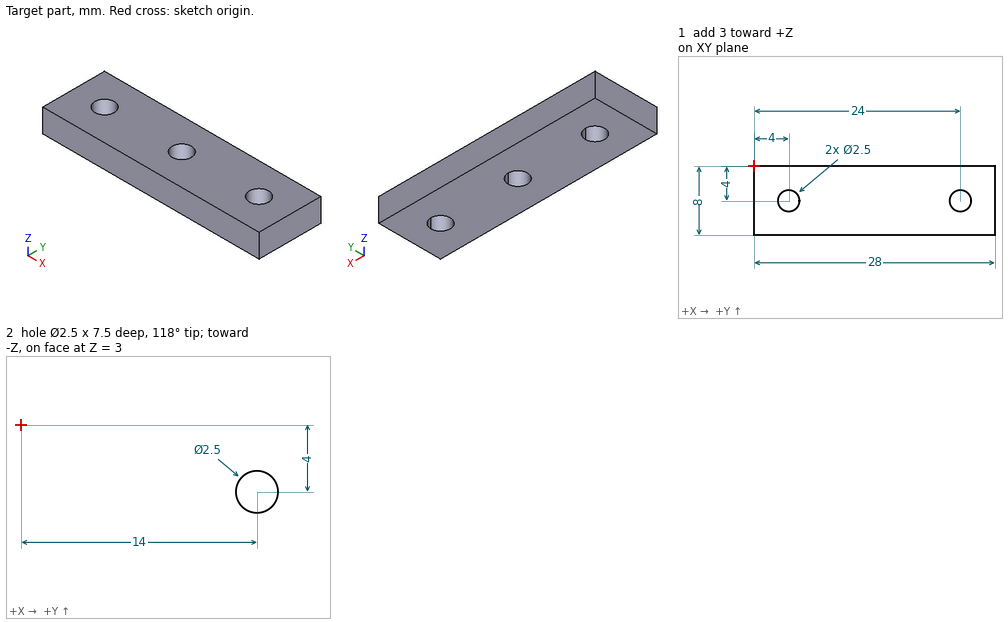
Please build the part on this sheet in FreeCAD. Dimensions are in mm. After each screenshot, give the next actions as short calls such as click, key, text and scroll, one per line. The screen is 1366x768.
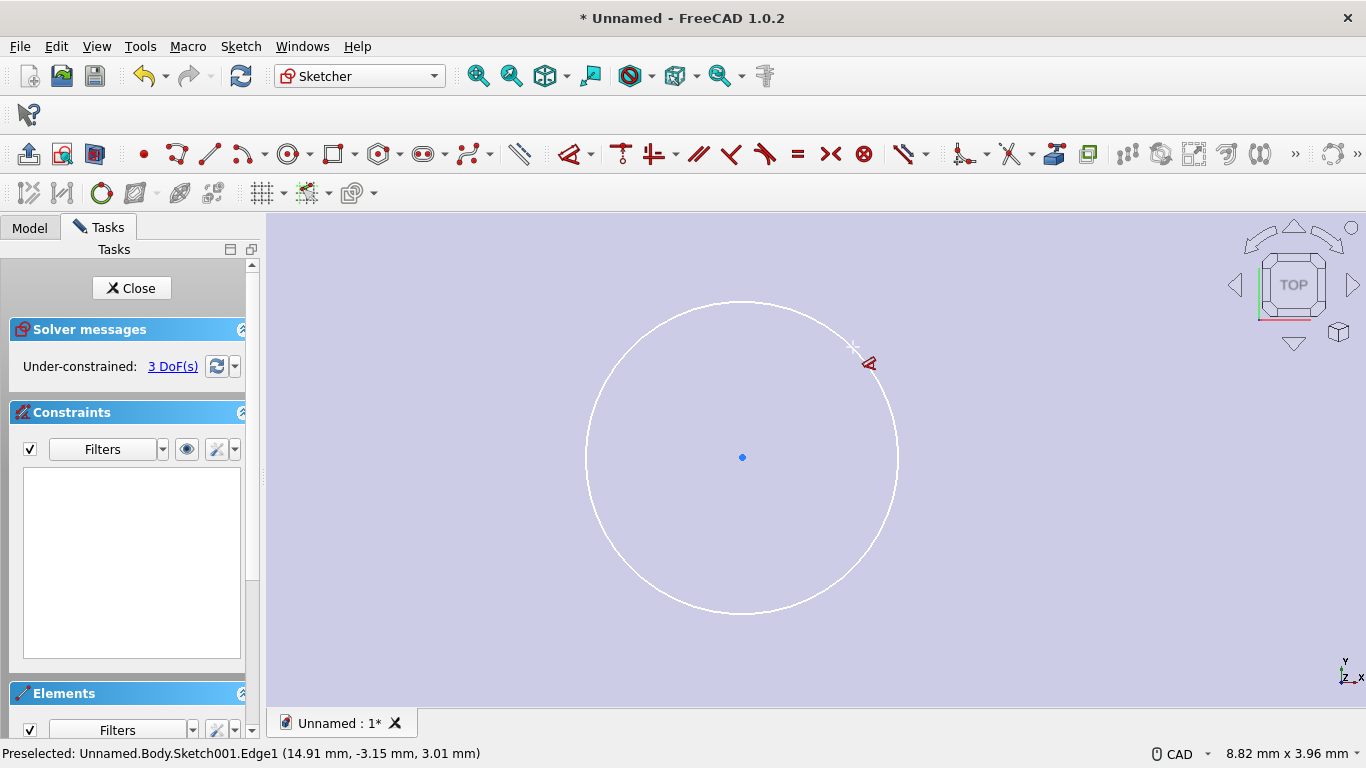
click(852, 347)
click(875, 324)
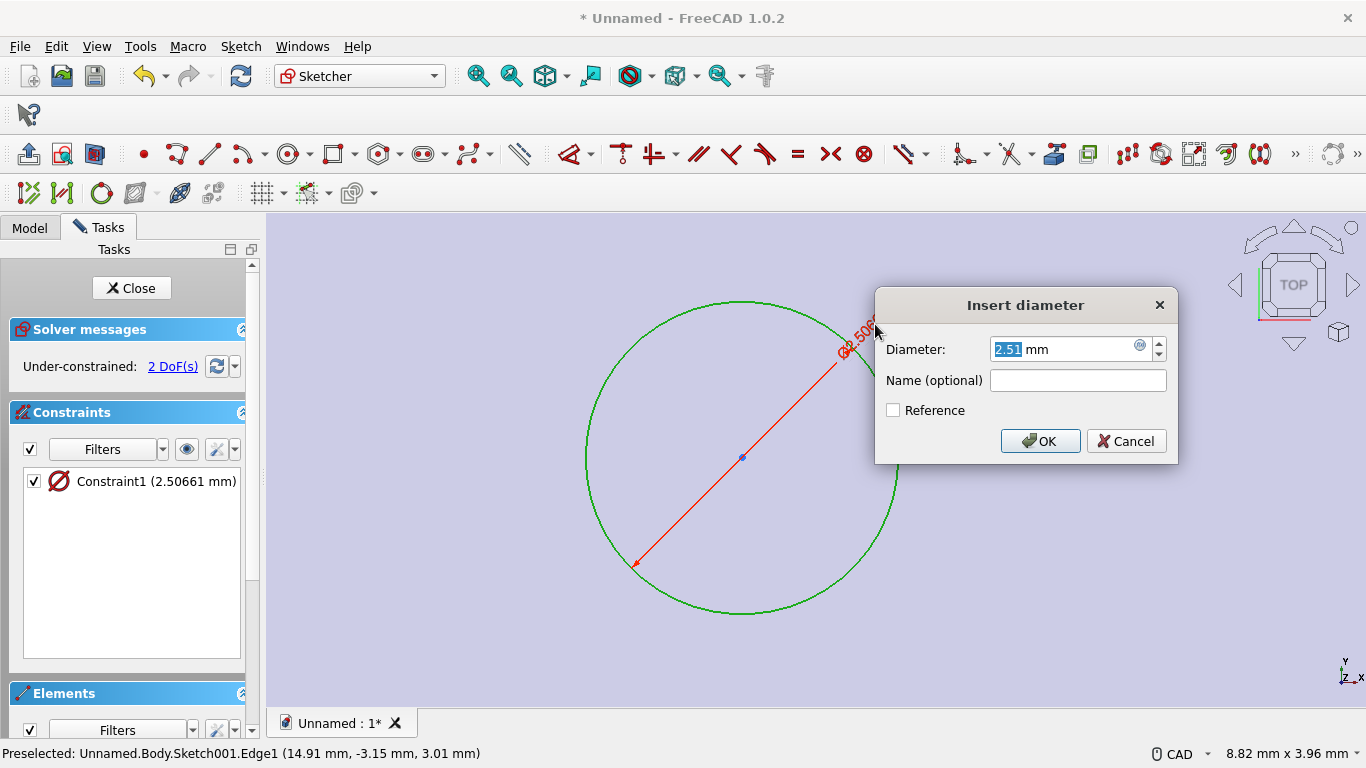
text(2.5)
key(Return)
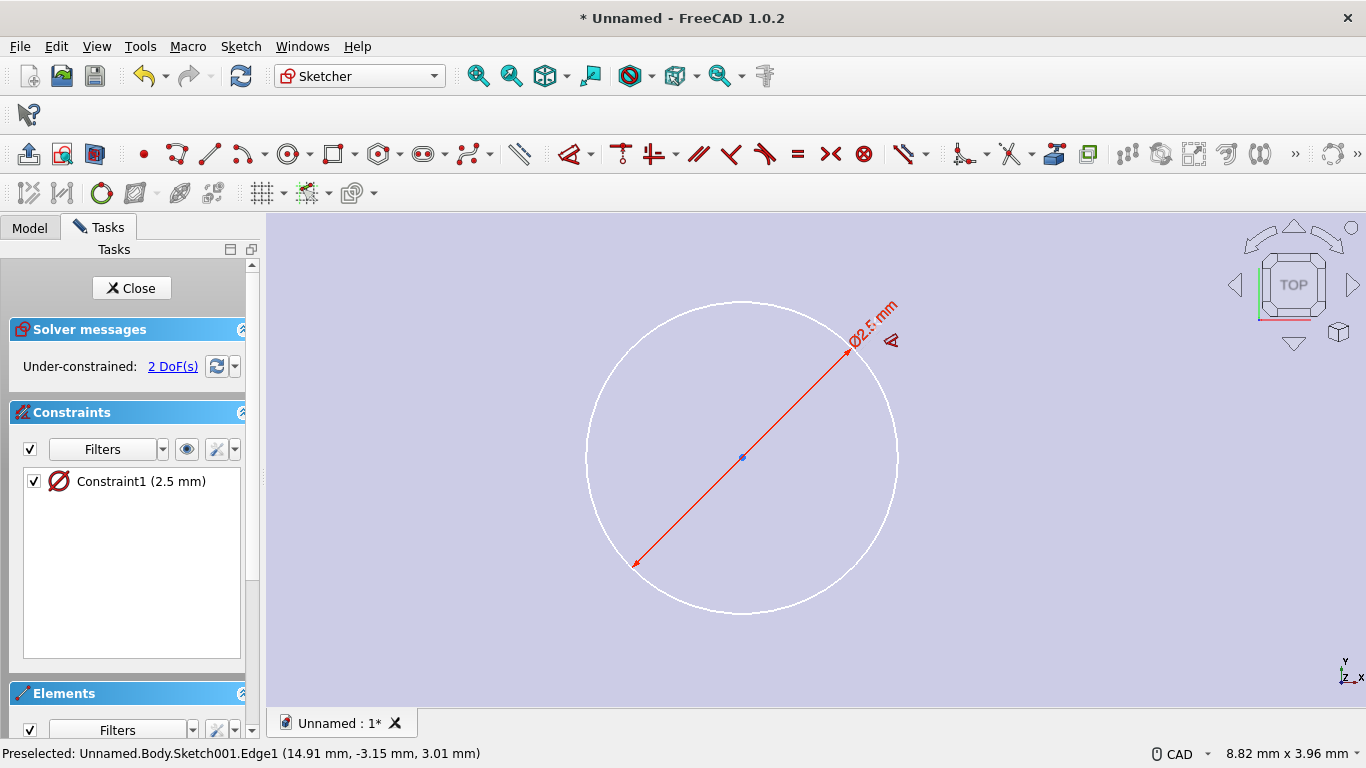
click(742, 458)
click(776, 350)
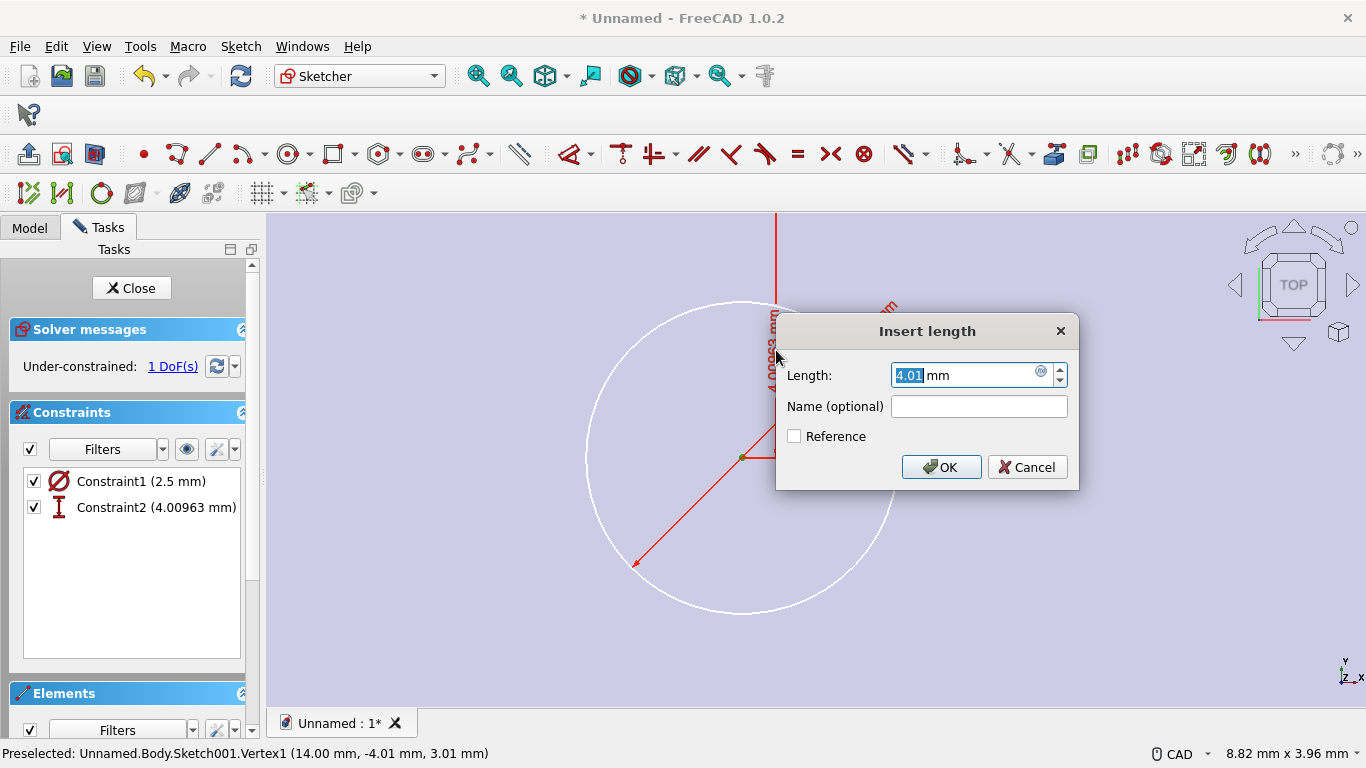
text(4)
key(Return)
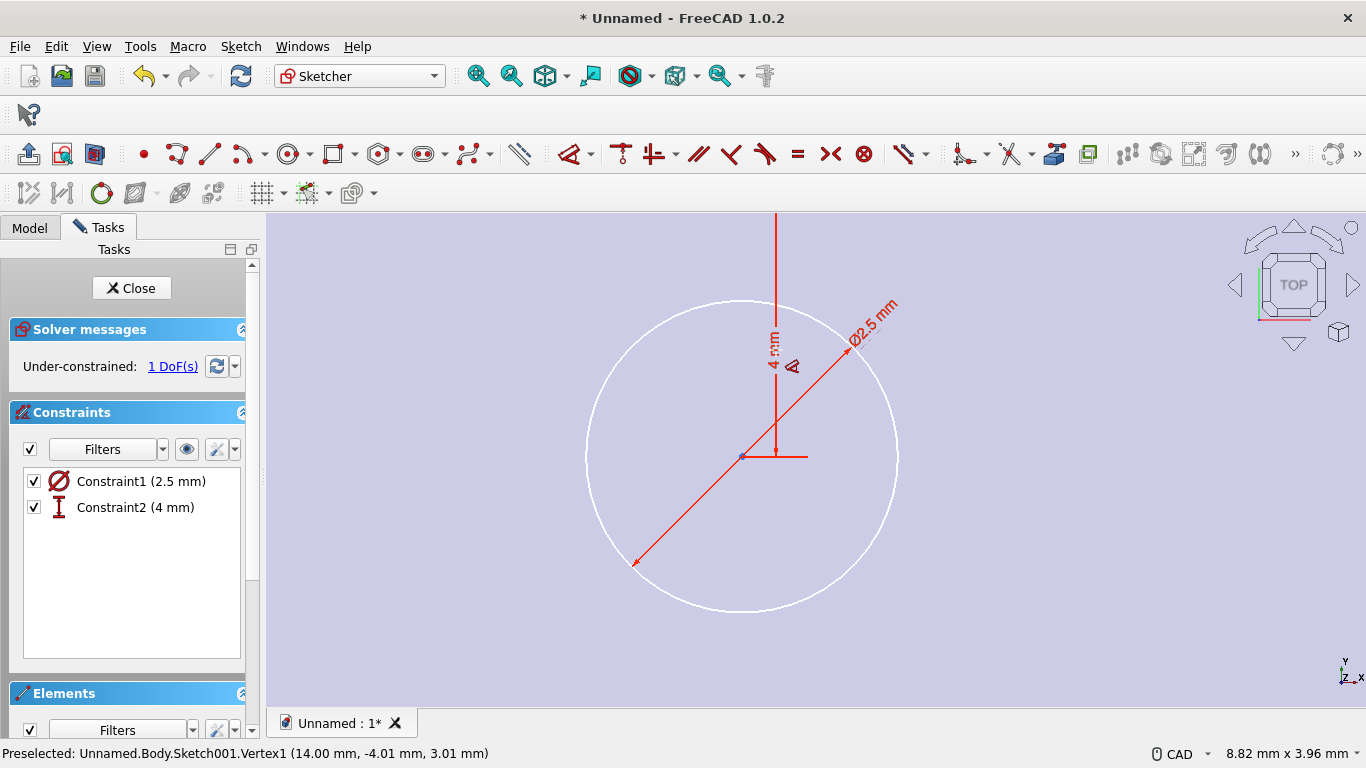
click(742, 457)
click(518, 491)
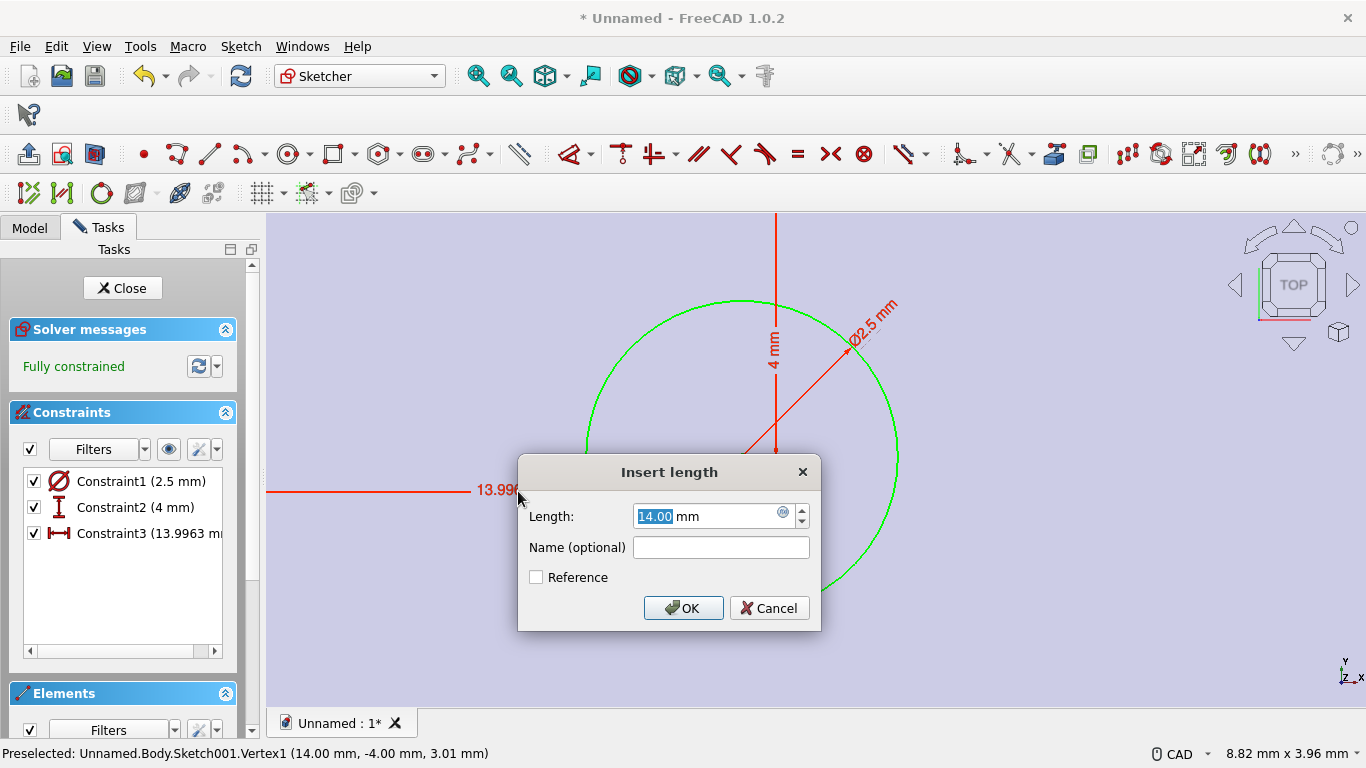
text(14)
key(Return)
key(Escape)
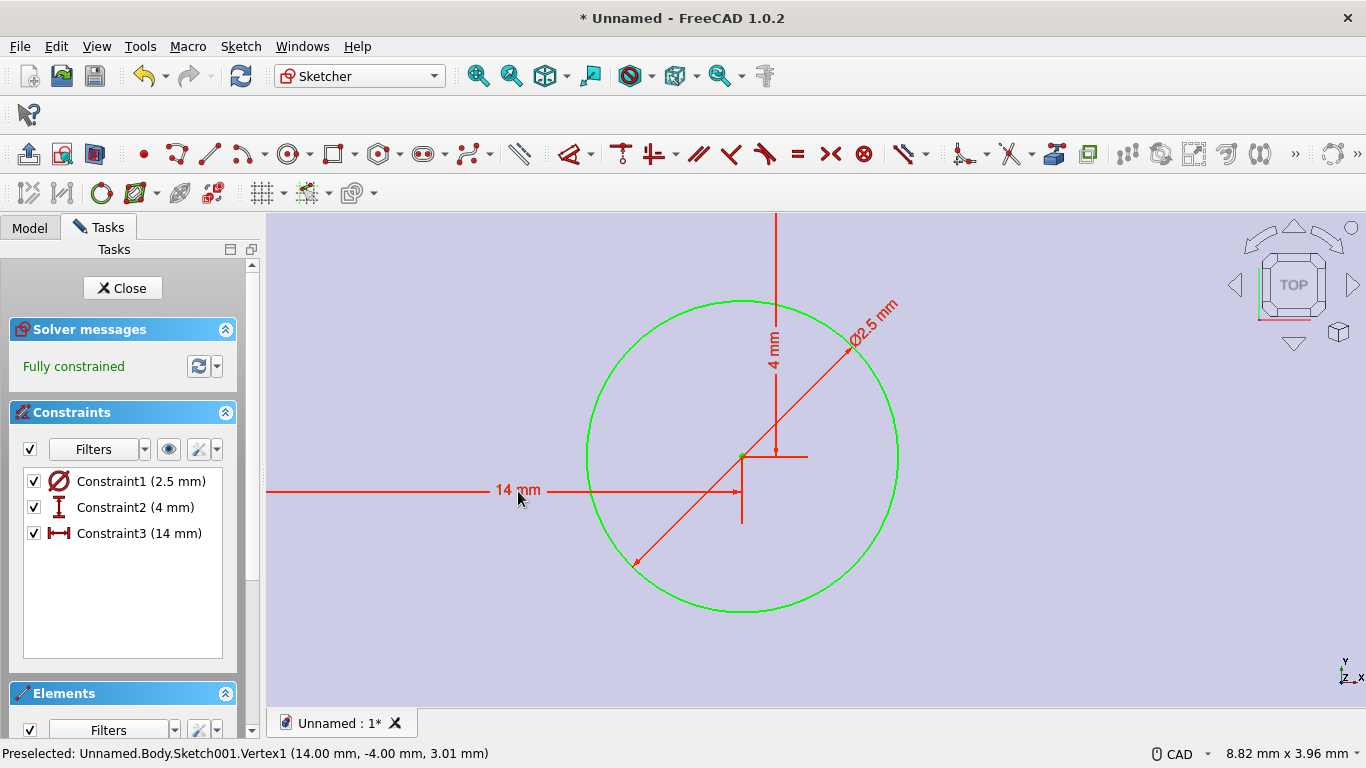
click(123, 288)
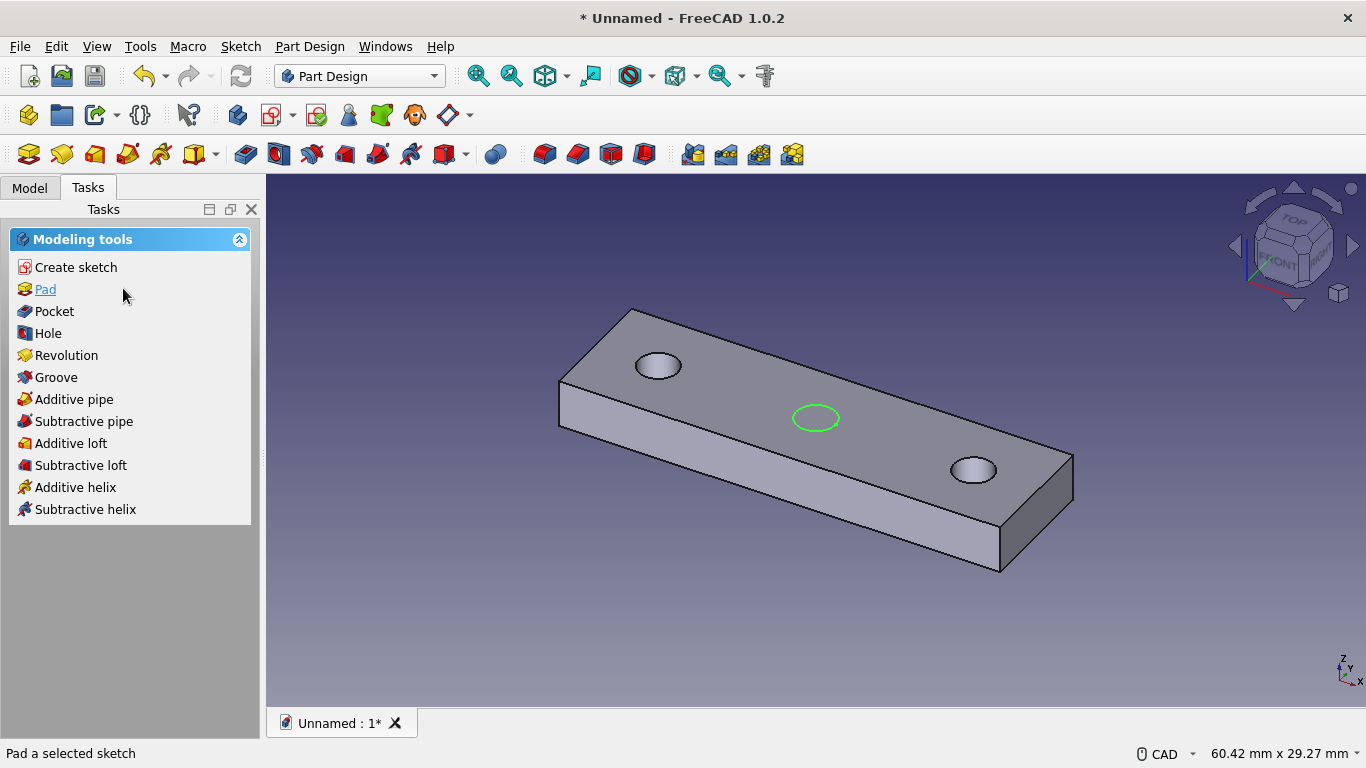
click(279, 154)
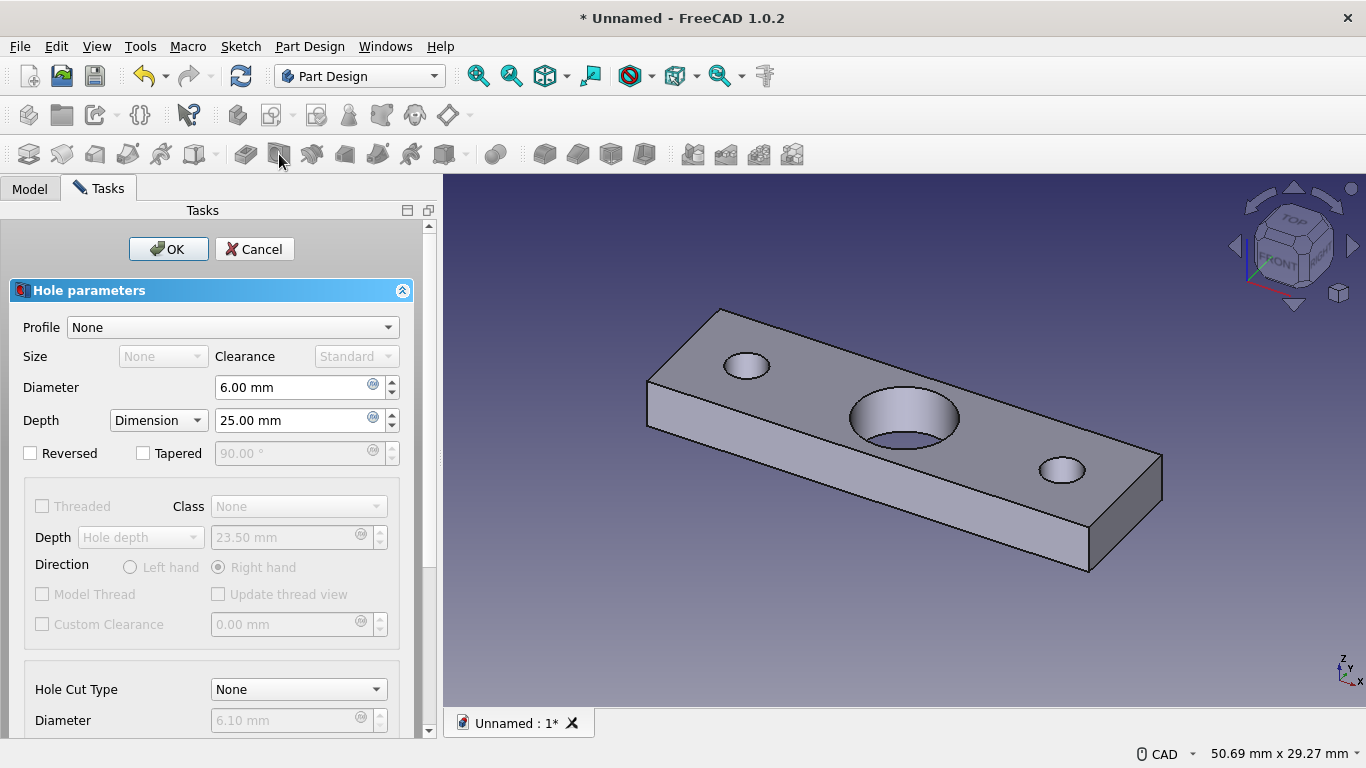
triple_click(300, 388)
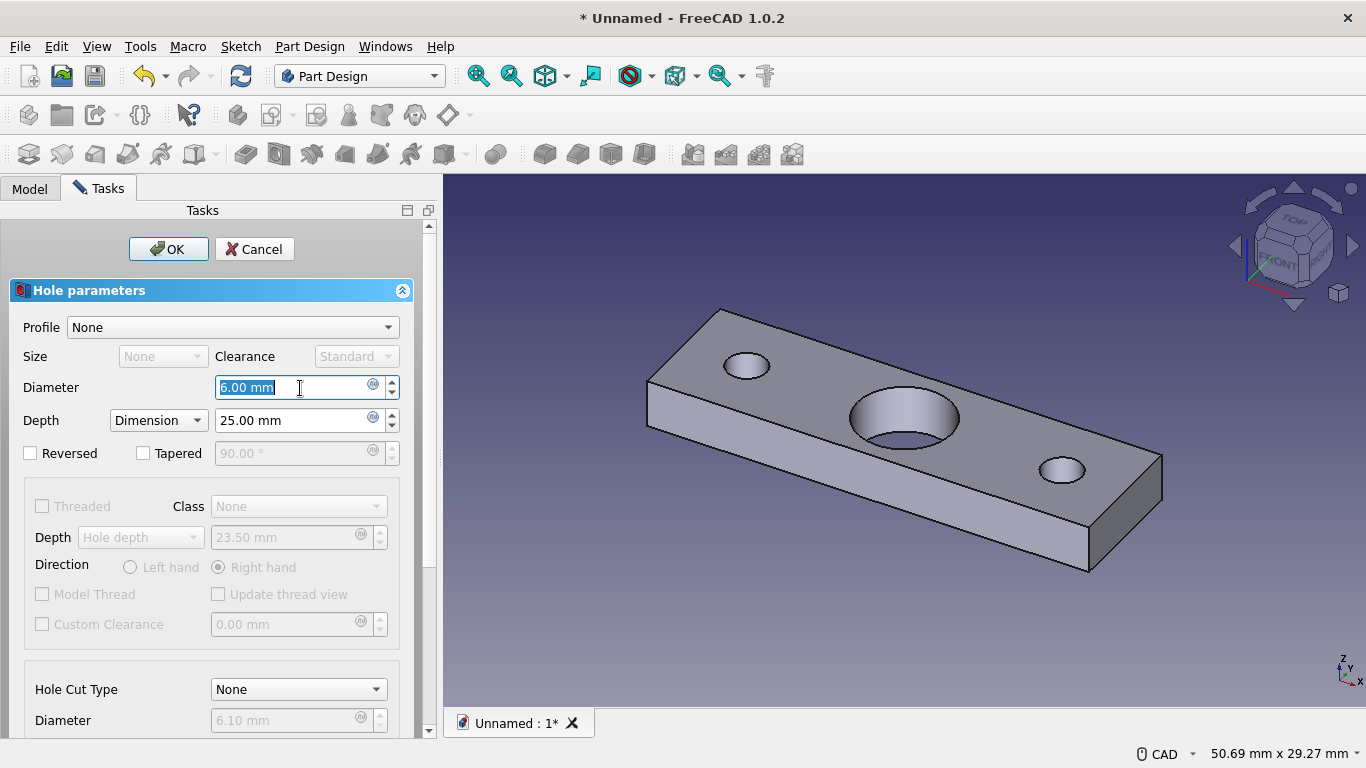
text(2.5)
key(Tab)